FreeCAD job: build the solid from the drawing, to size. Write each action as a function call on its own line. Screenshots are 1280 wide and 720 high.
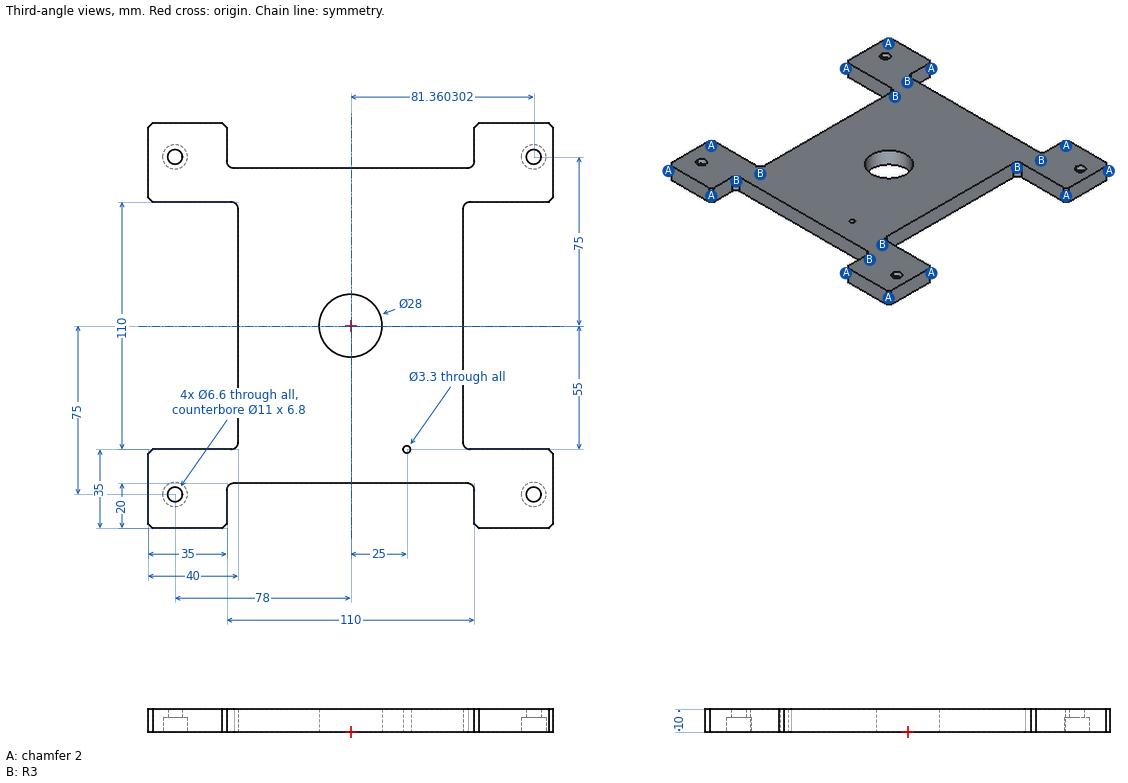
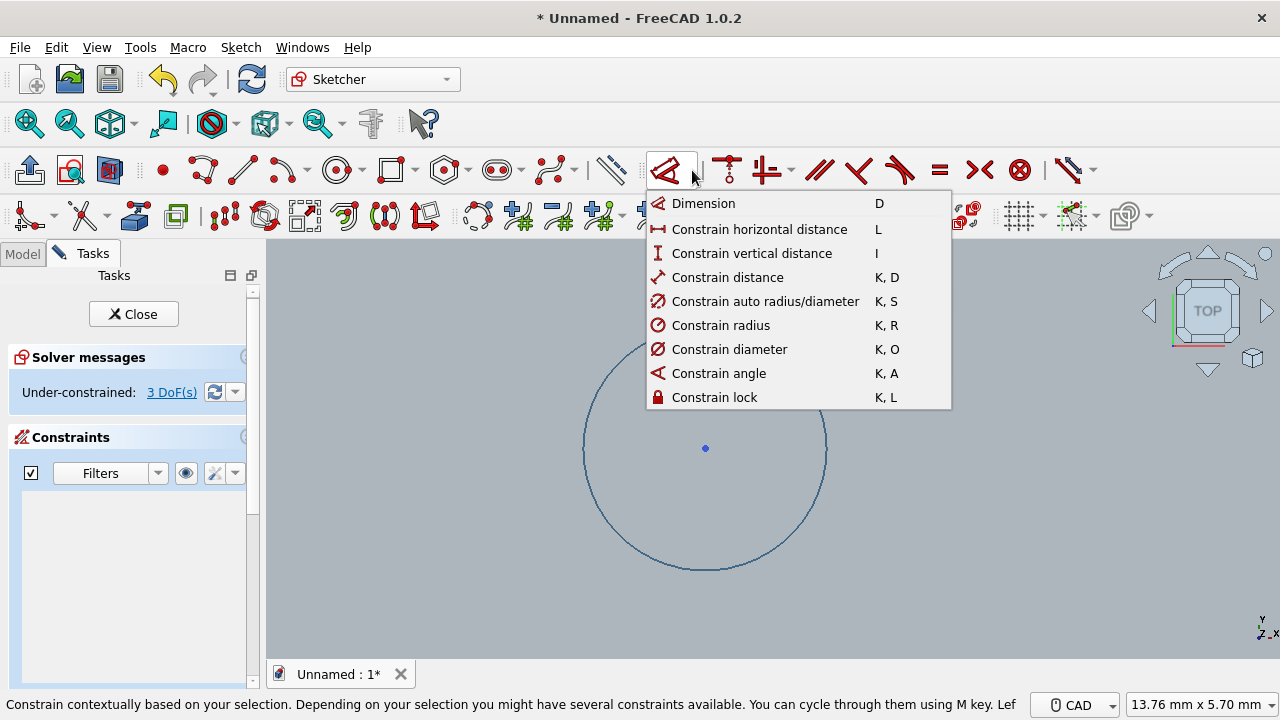
click(799, 349)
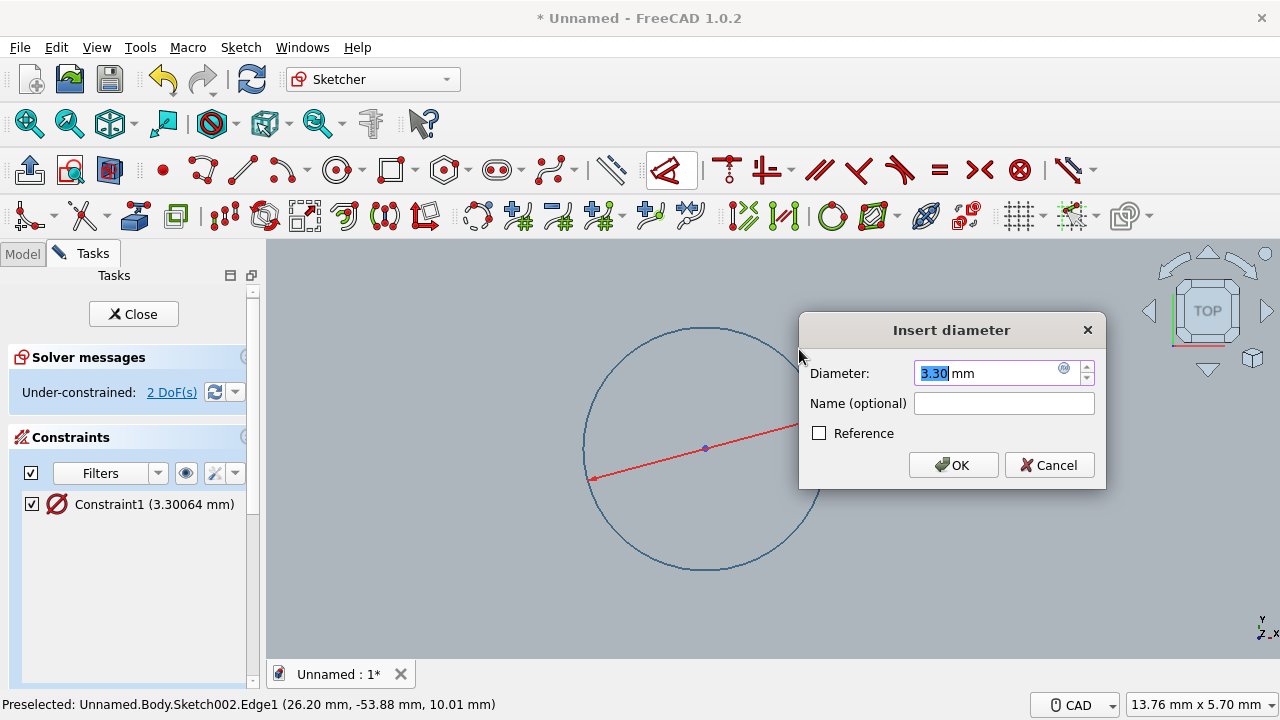
text(3.3)
key(Return)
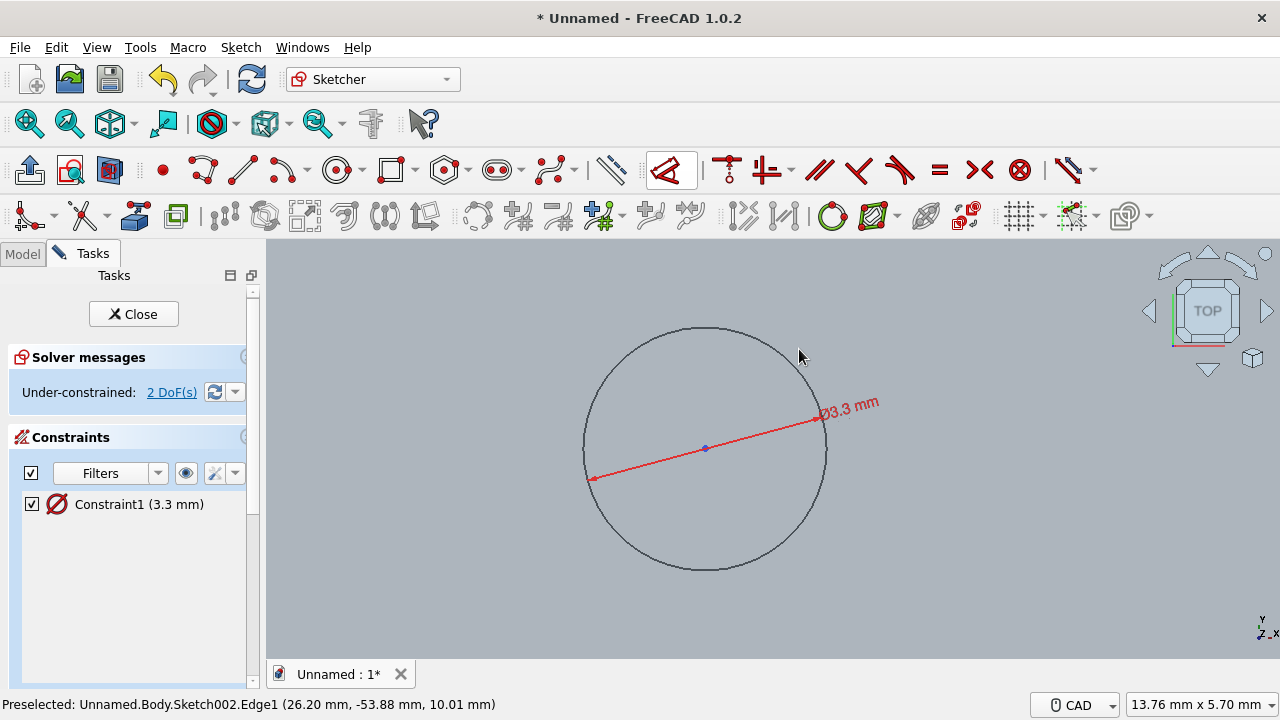
click(705, 449)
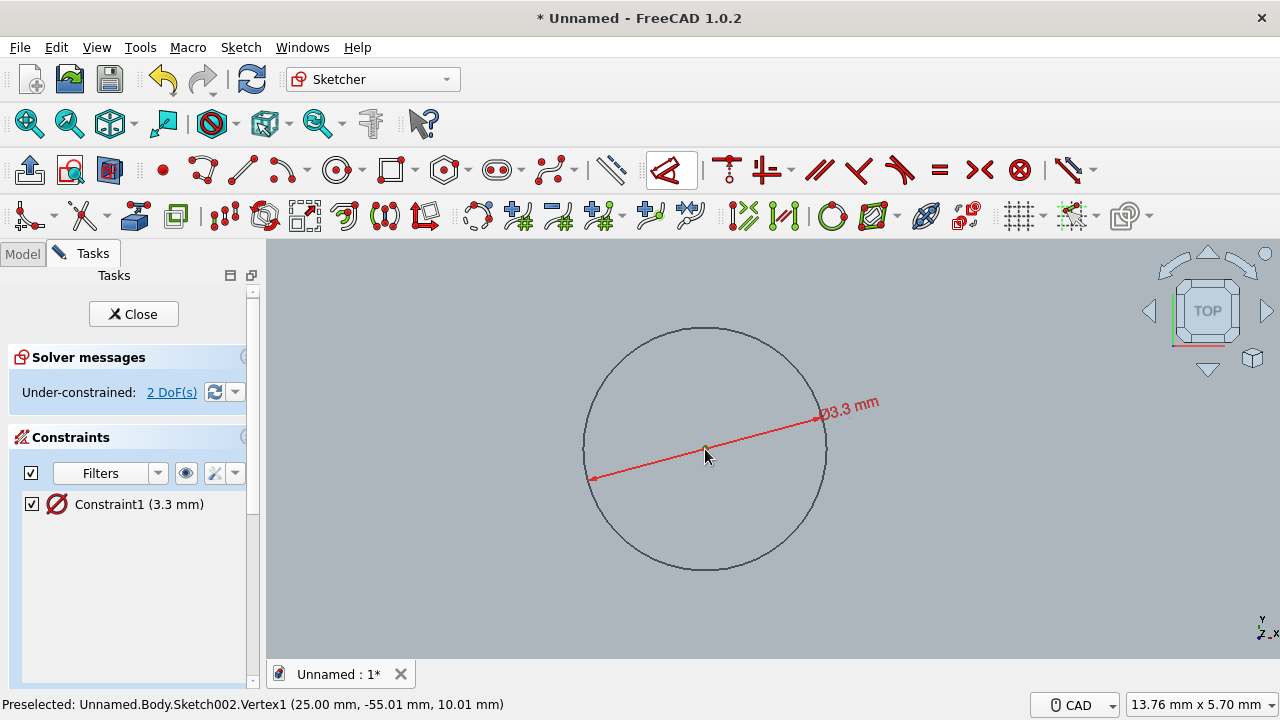
click(692, 170)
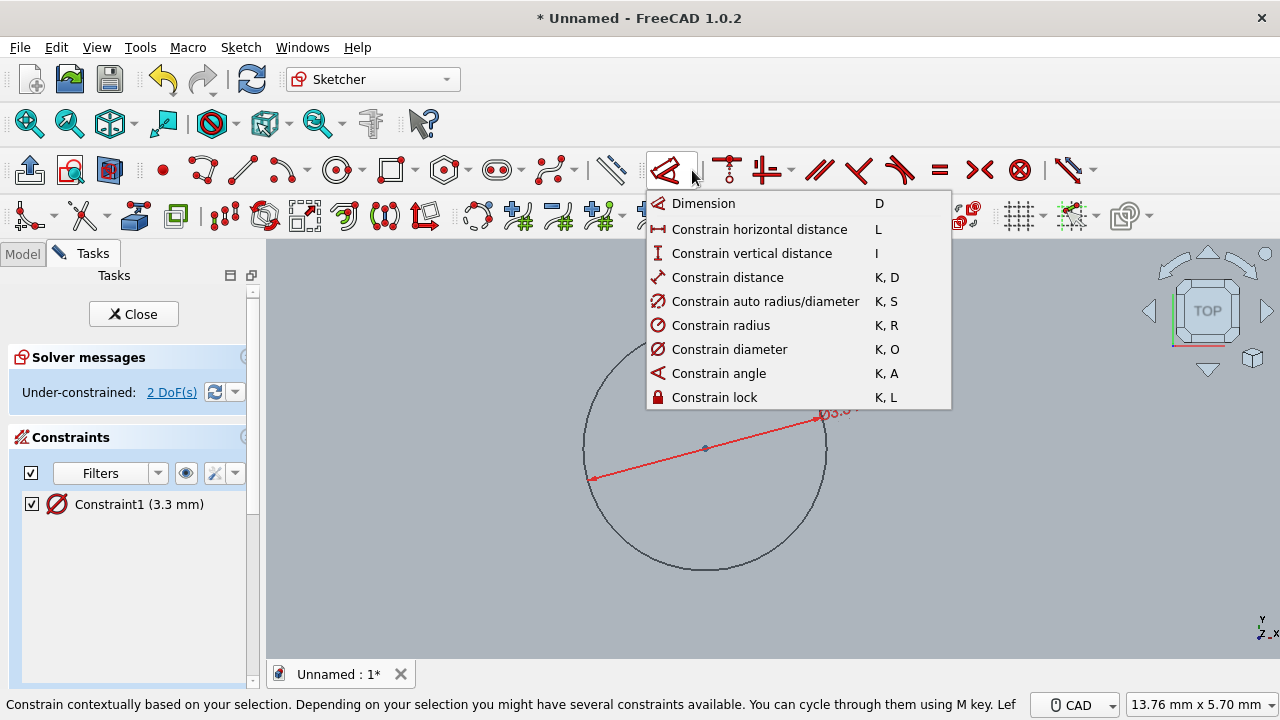
click(799, 229)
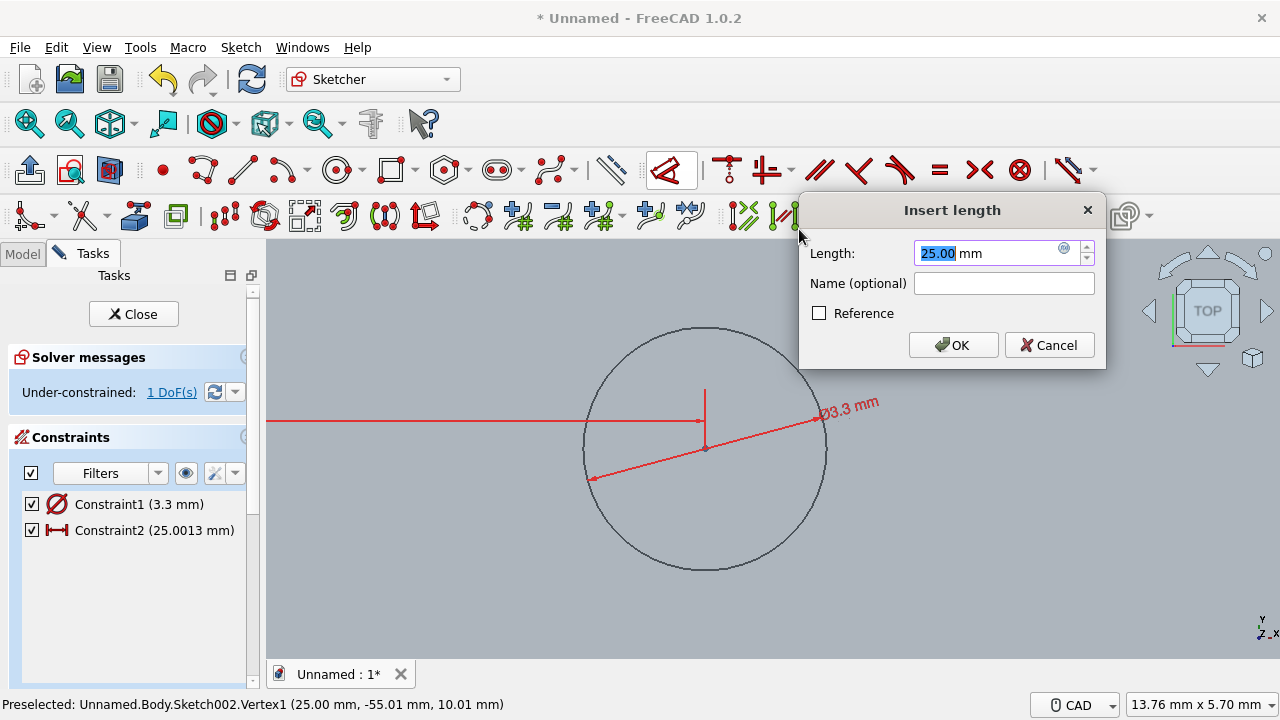
text(25)
key(Return)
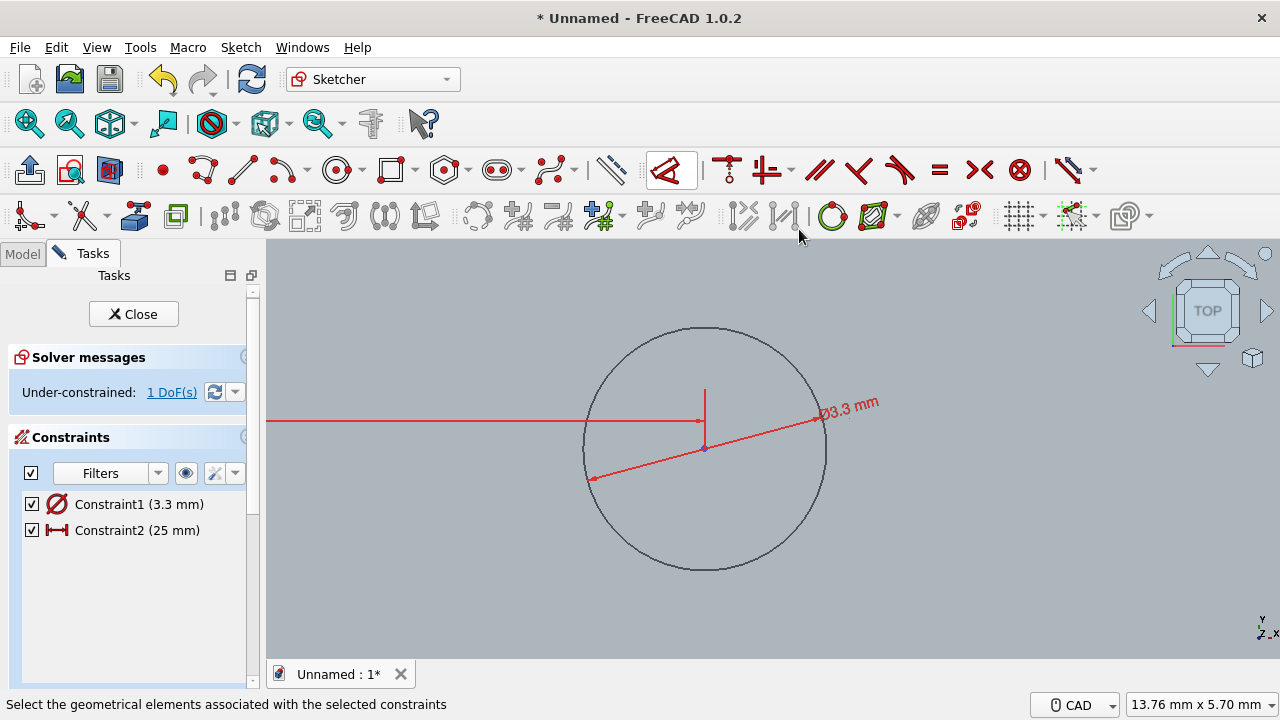
click(705, 449)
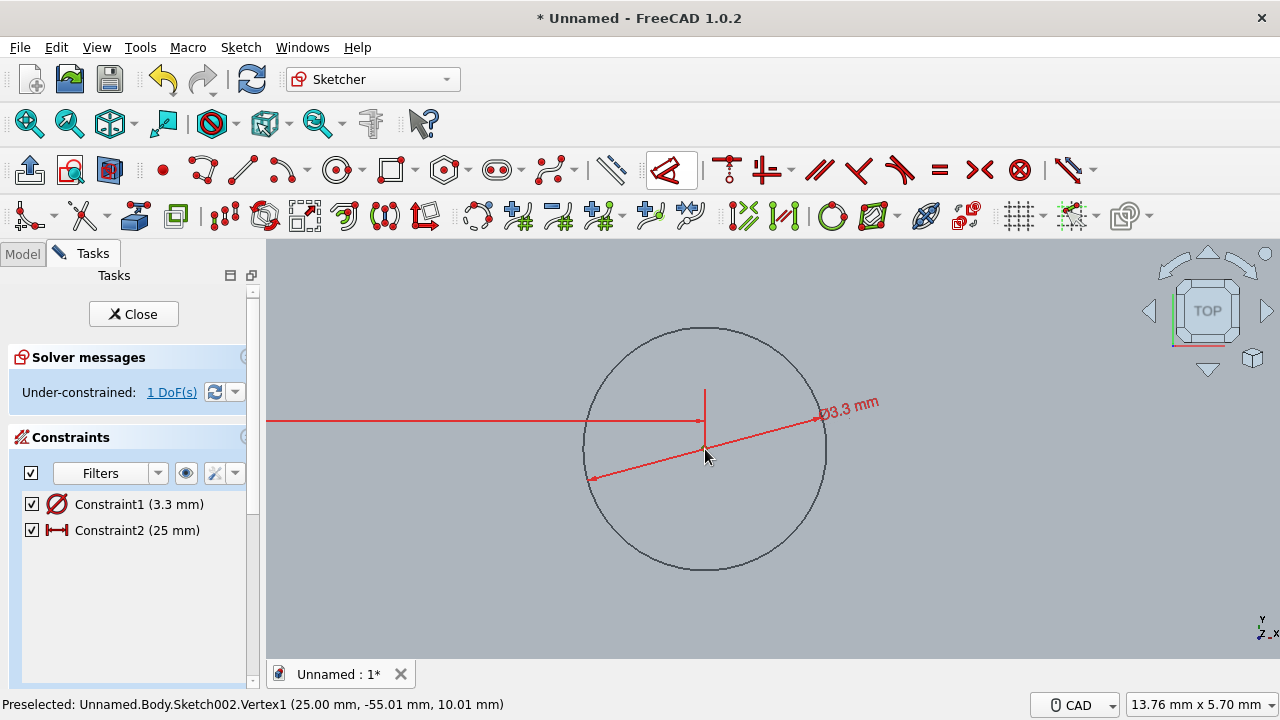
key(i)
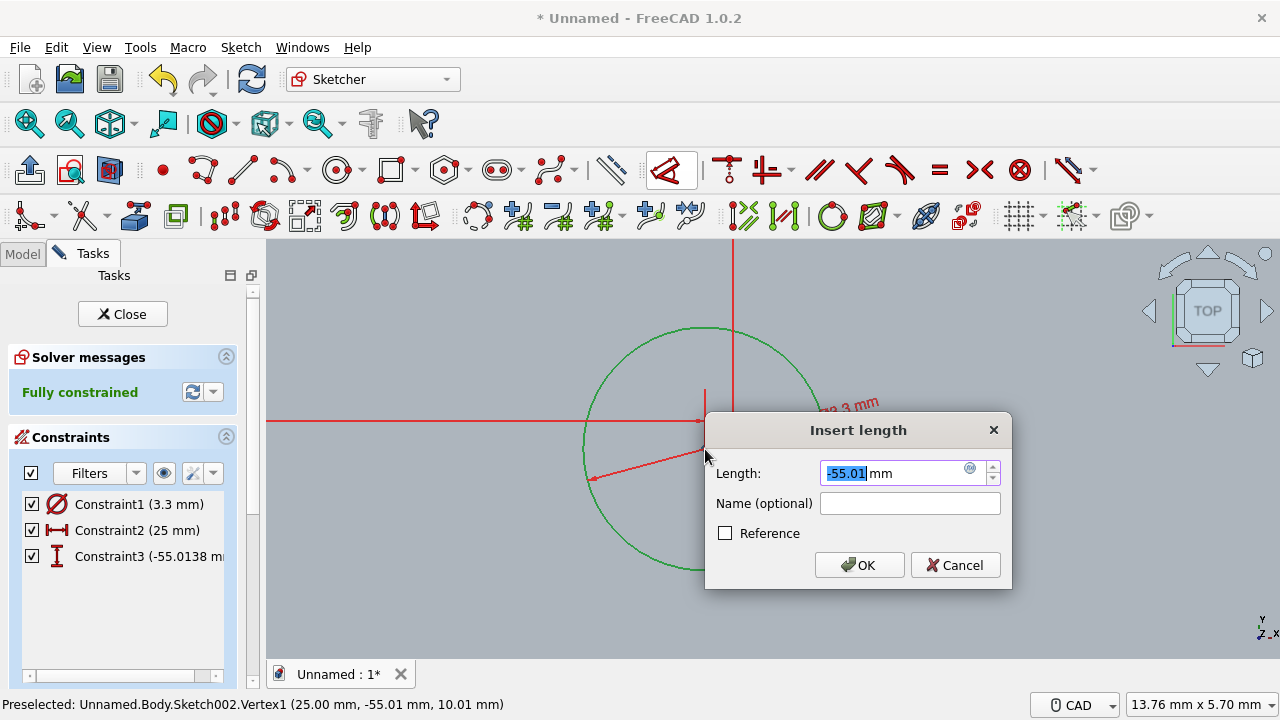
text(-55)
key(Return)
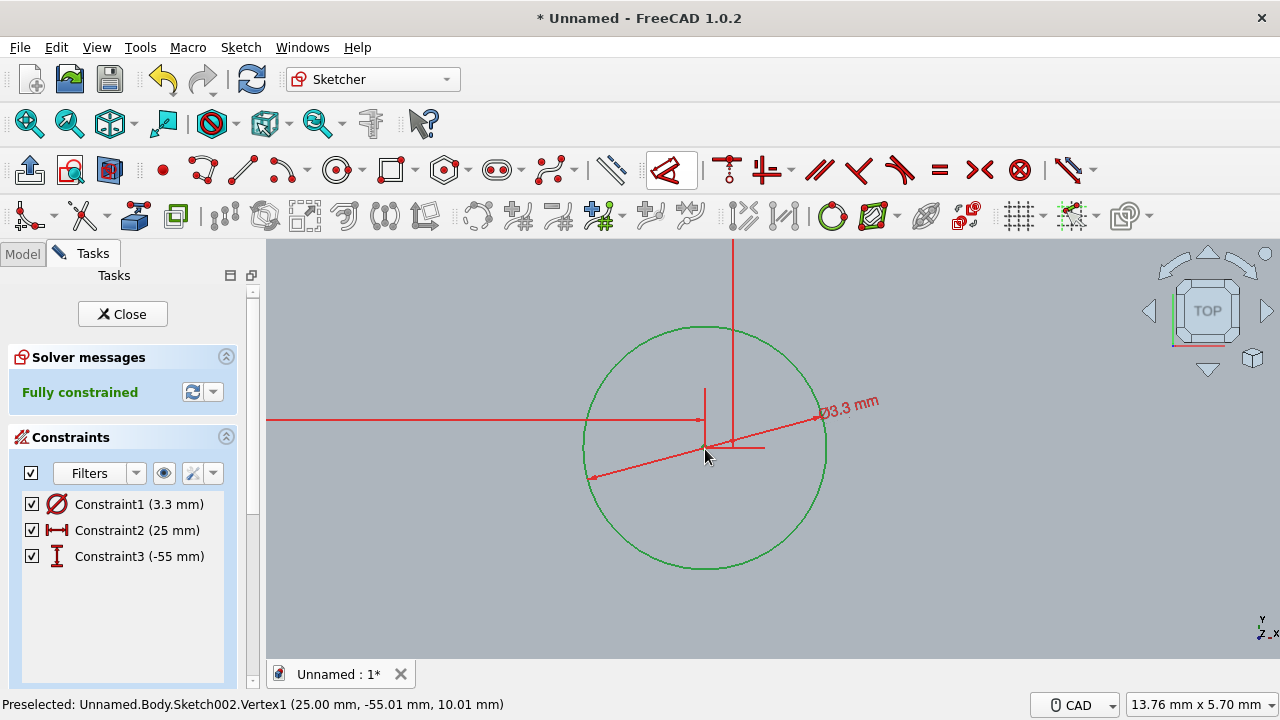
click(123, 314)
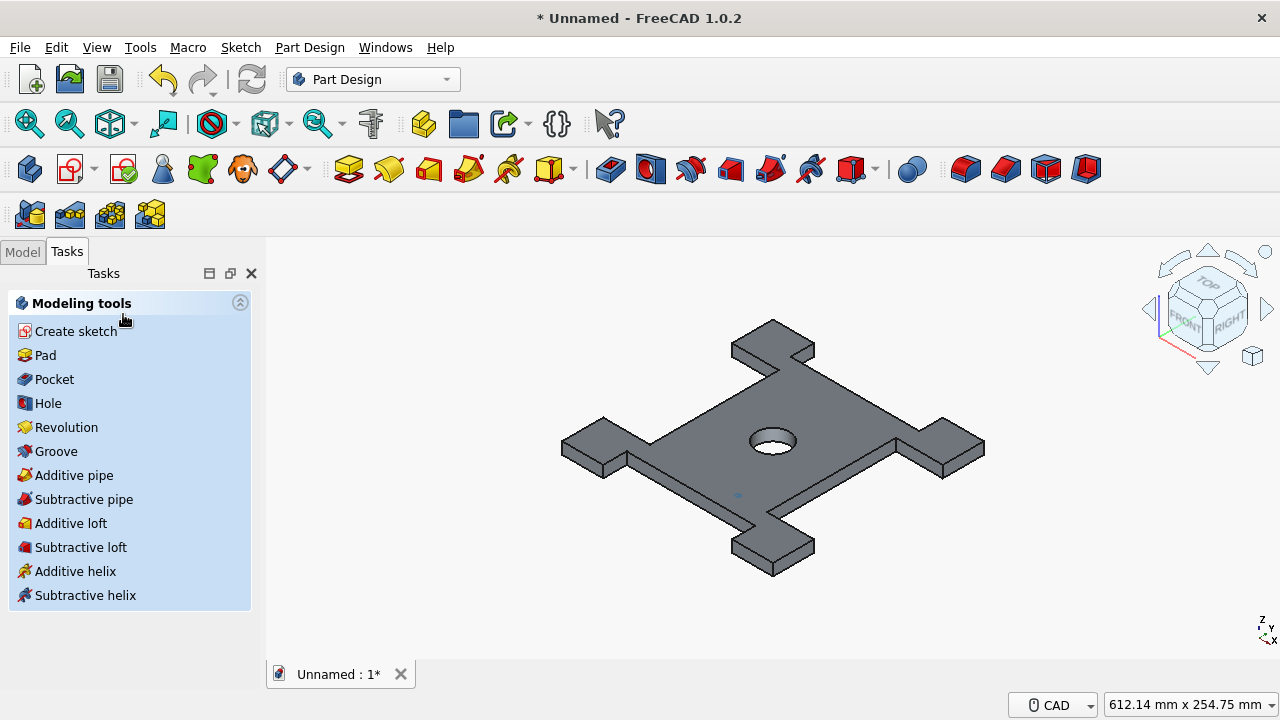
click(652, 170)